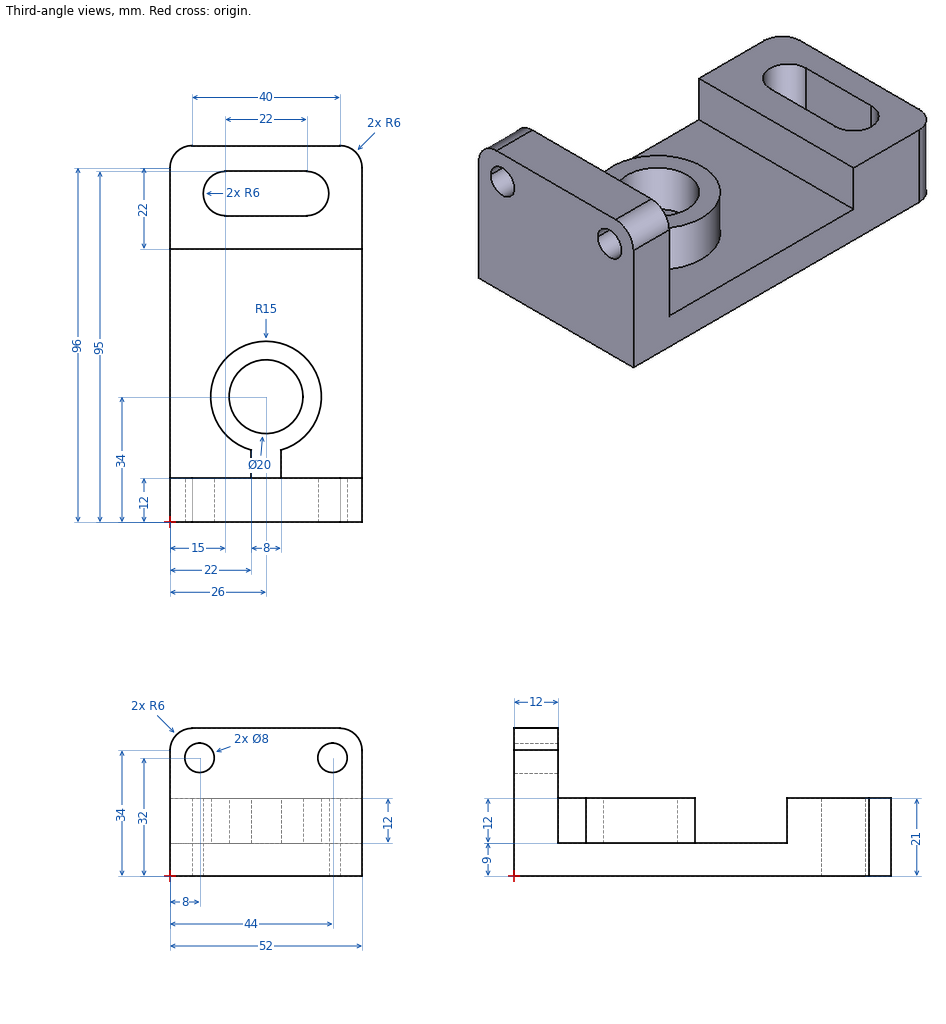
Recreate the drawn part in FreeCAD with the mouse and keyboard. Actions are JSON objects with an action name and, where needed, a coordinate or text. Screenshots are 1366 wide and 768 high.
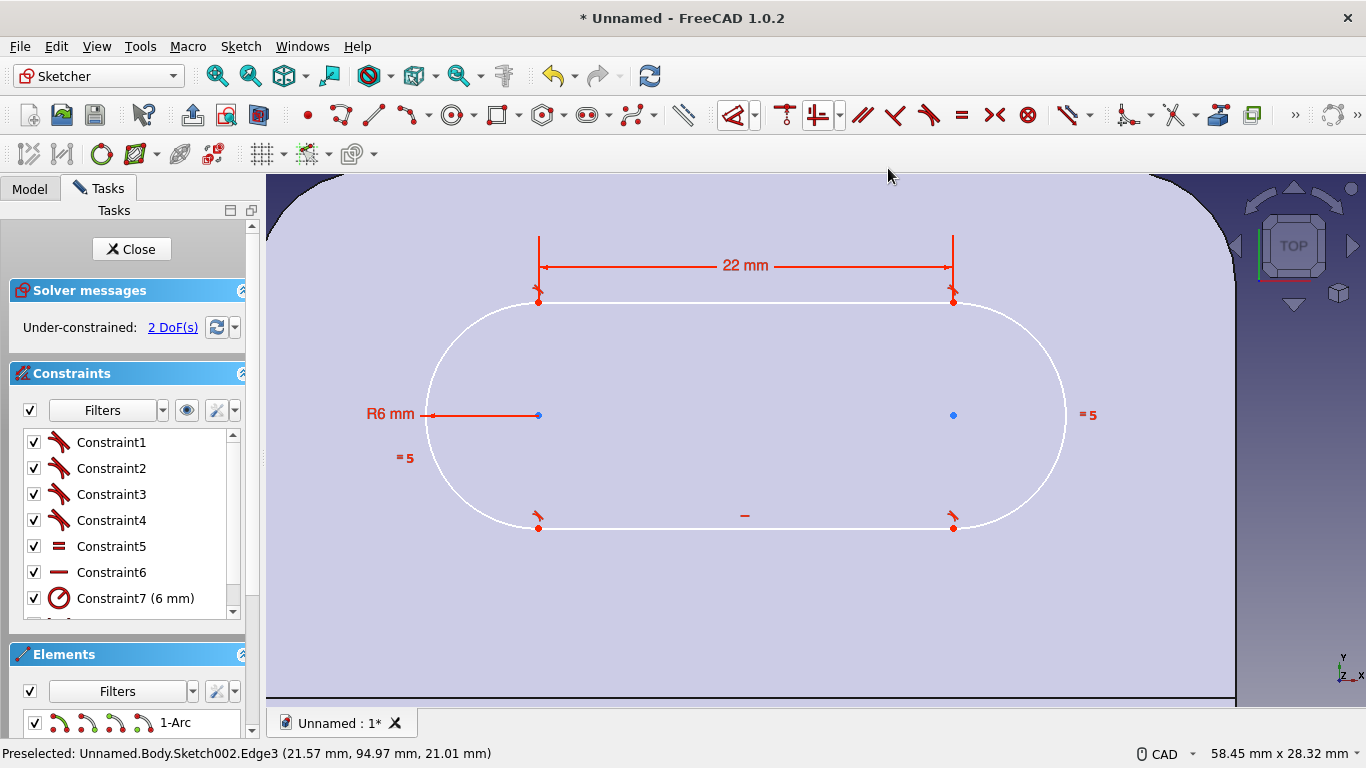
{"action": "left_click", "coordinate": [539, 303]}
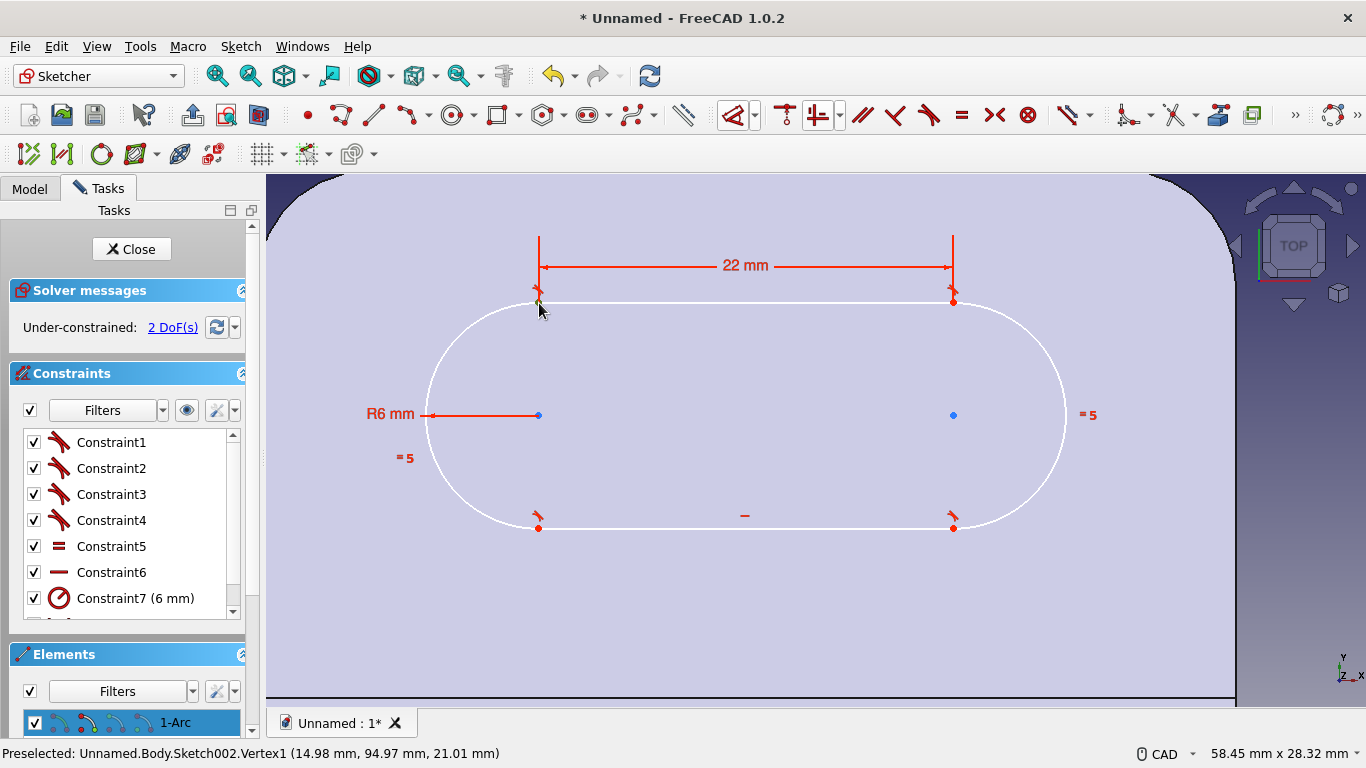
{"action": "key", "text": "l"}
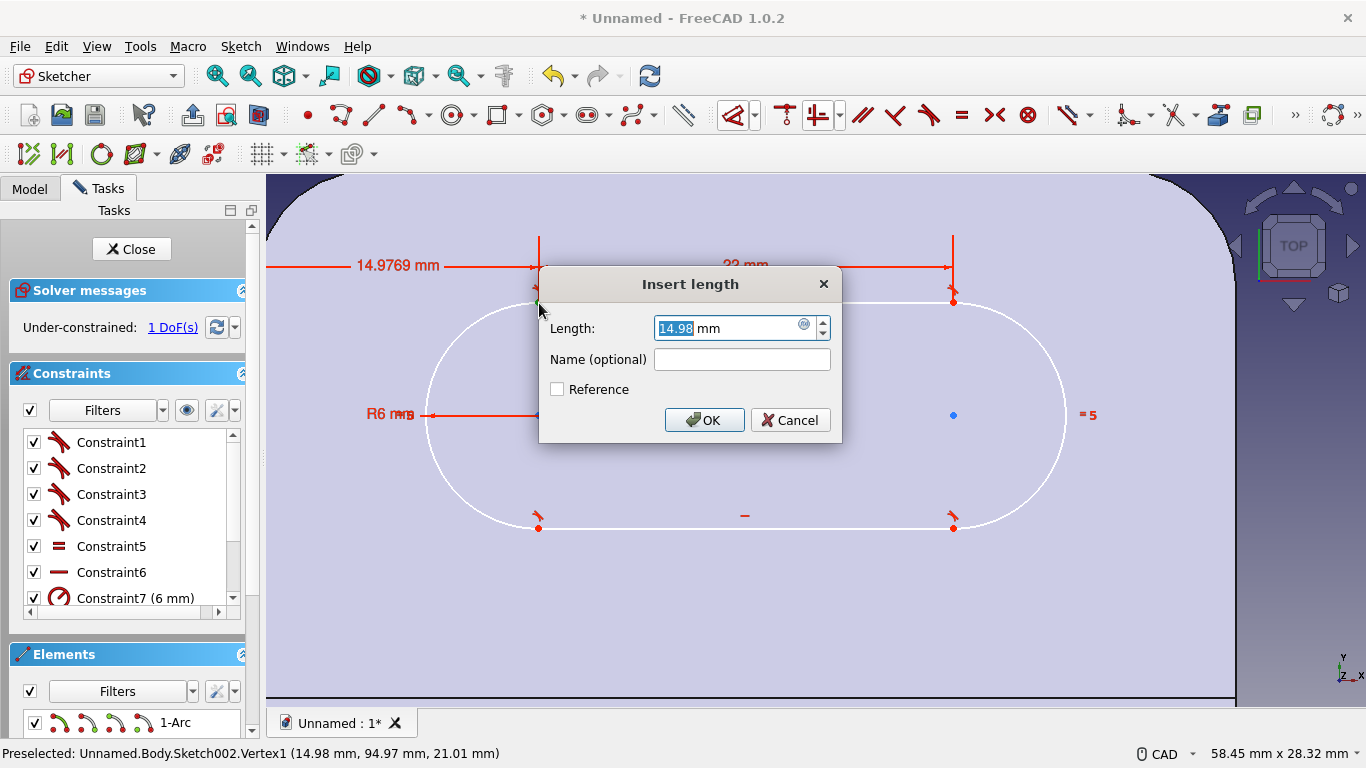
{"action": "type", "text": "15"}
{"action": "key", "text": "Return"}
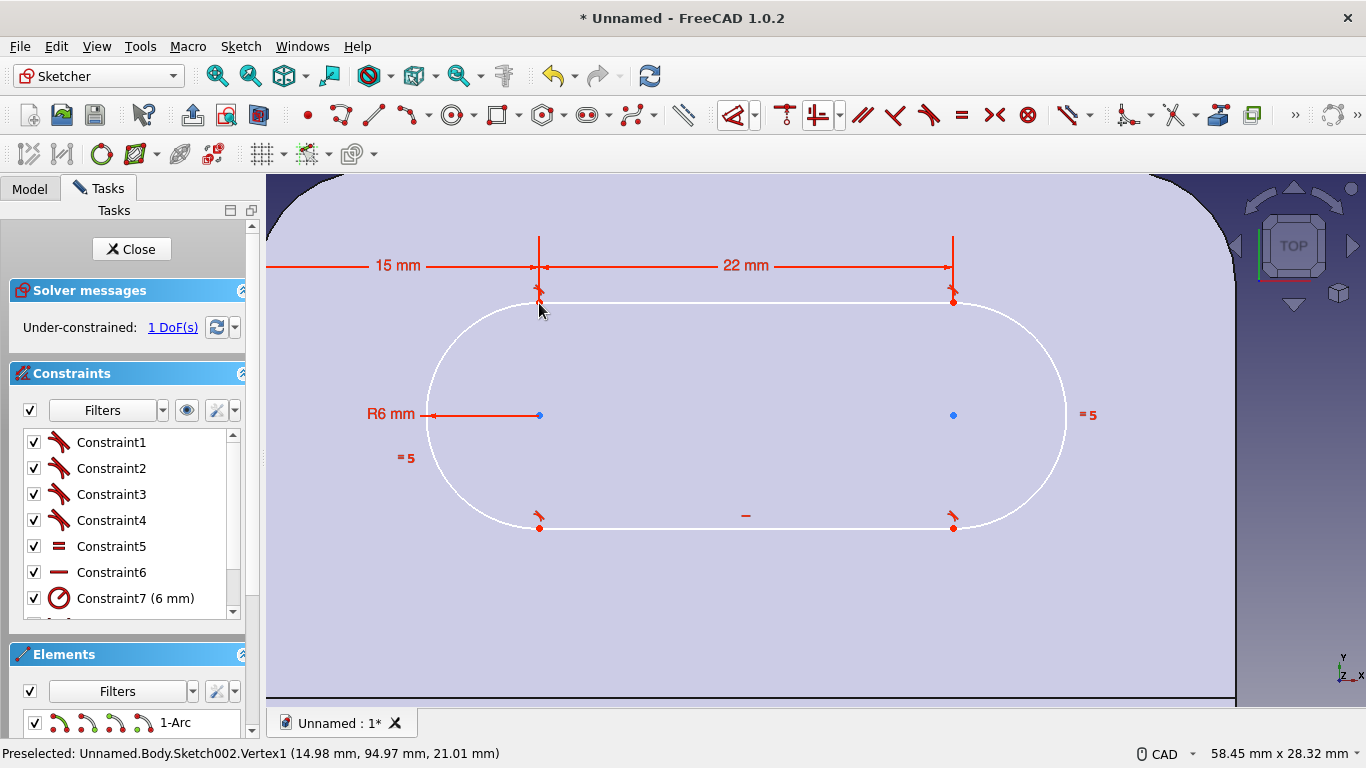
{"action": "left_click", "coordinate": [539, 303]}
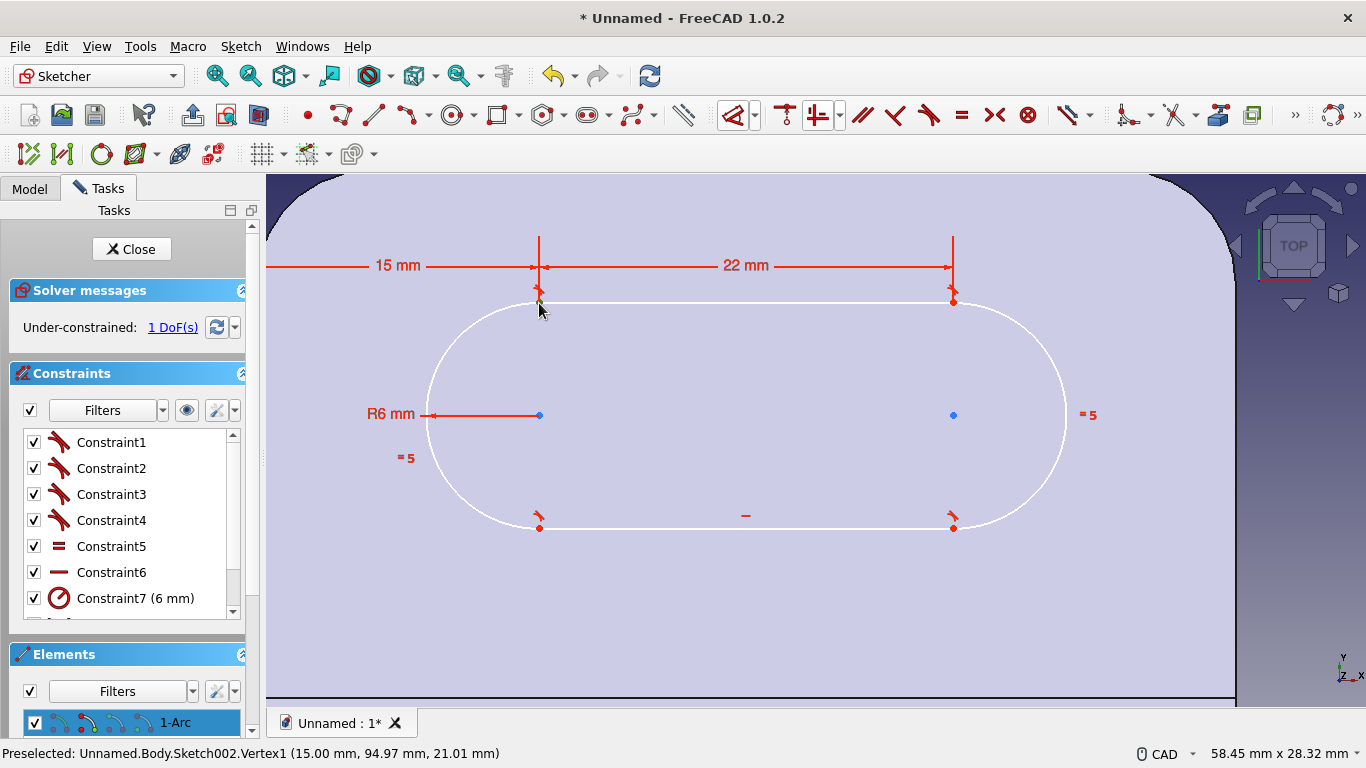
{"action": "key", "text": "i"}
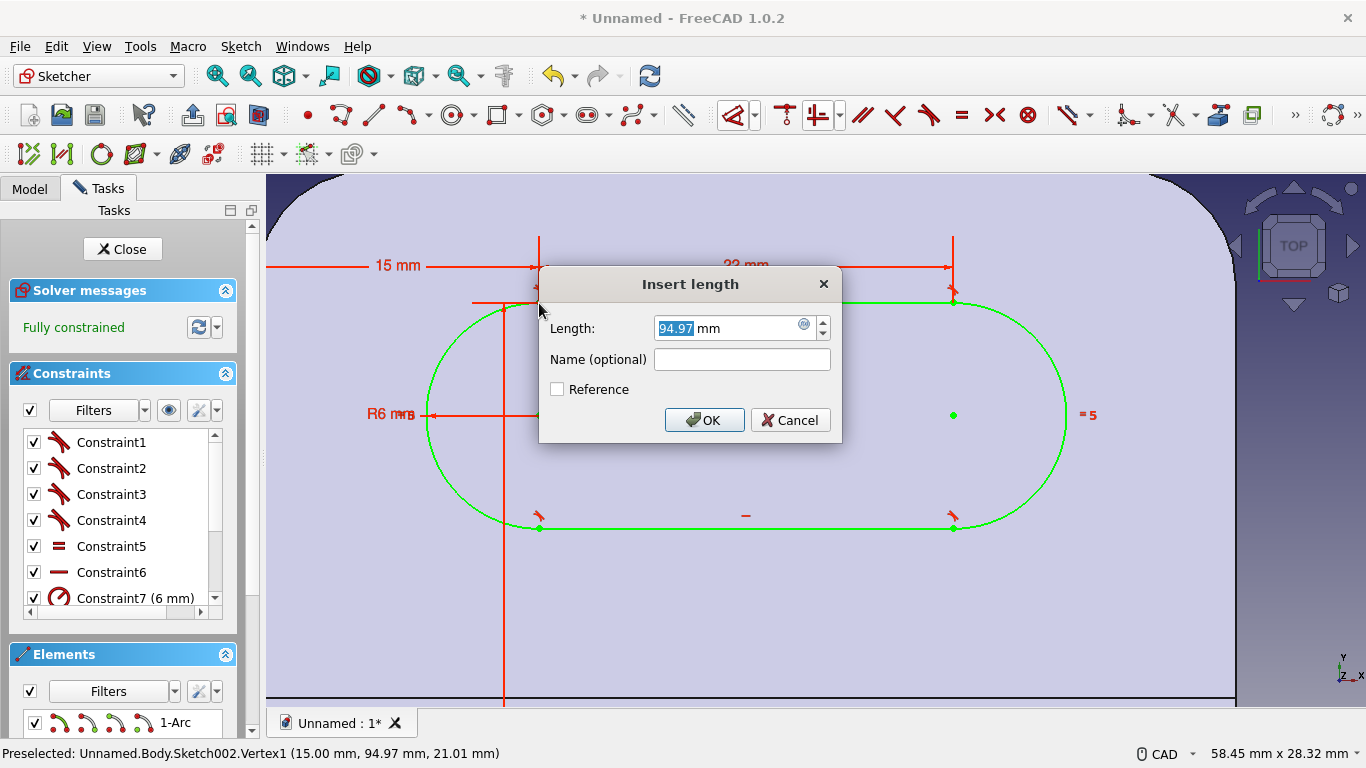
{"action": "type", "text": "95"}
{"action": "key", "text": "Return"}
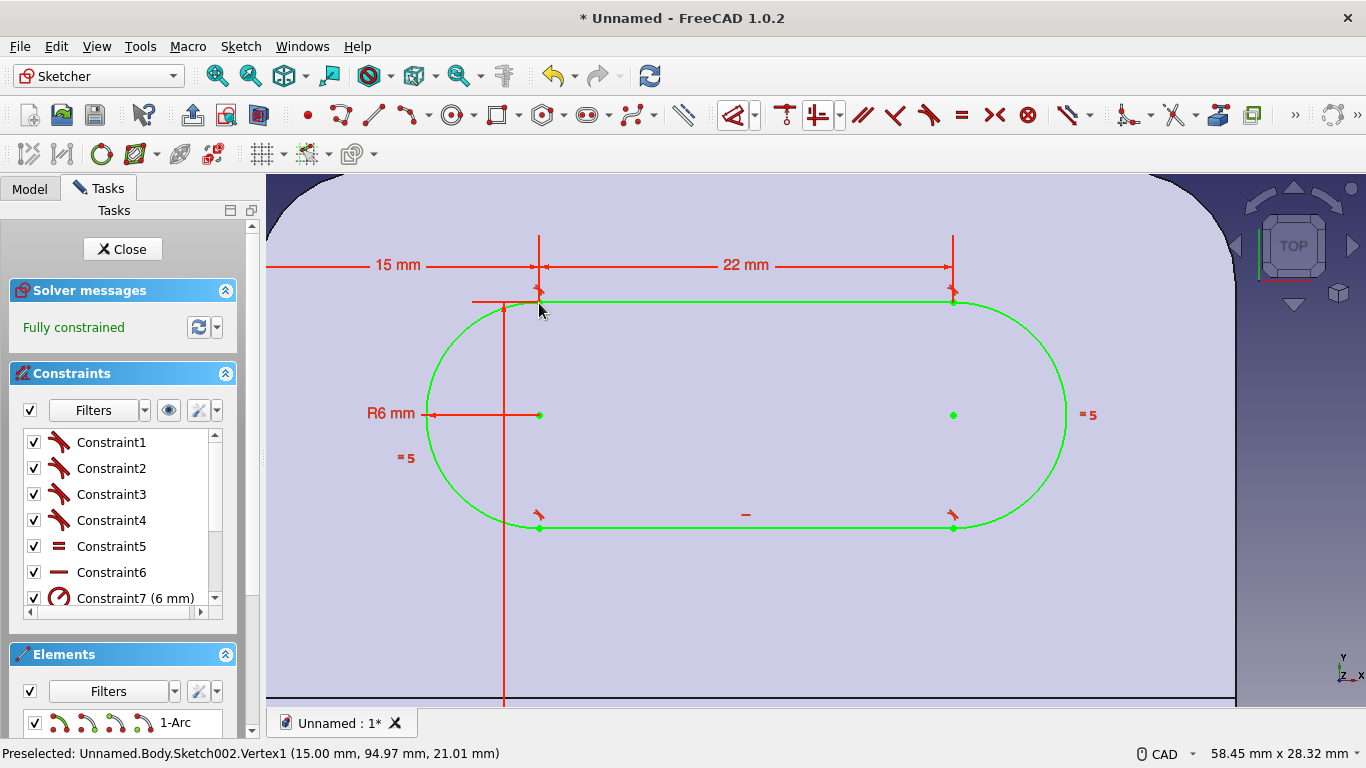
{"action": "left_click", "coordinate": [123, 249]}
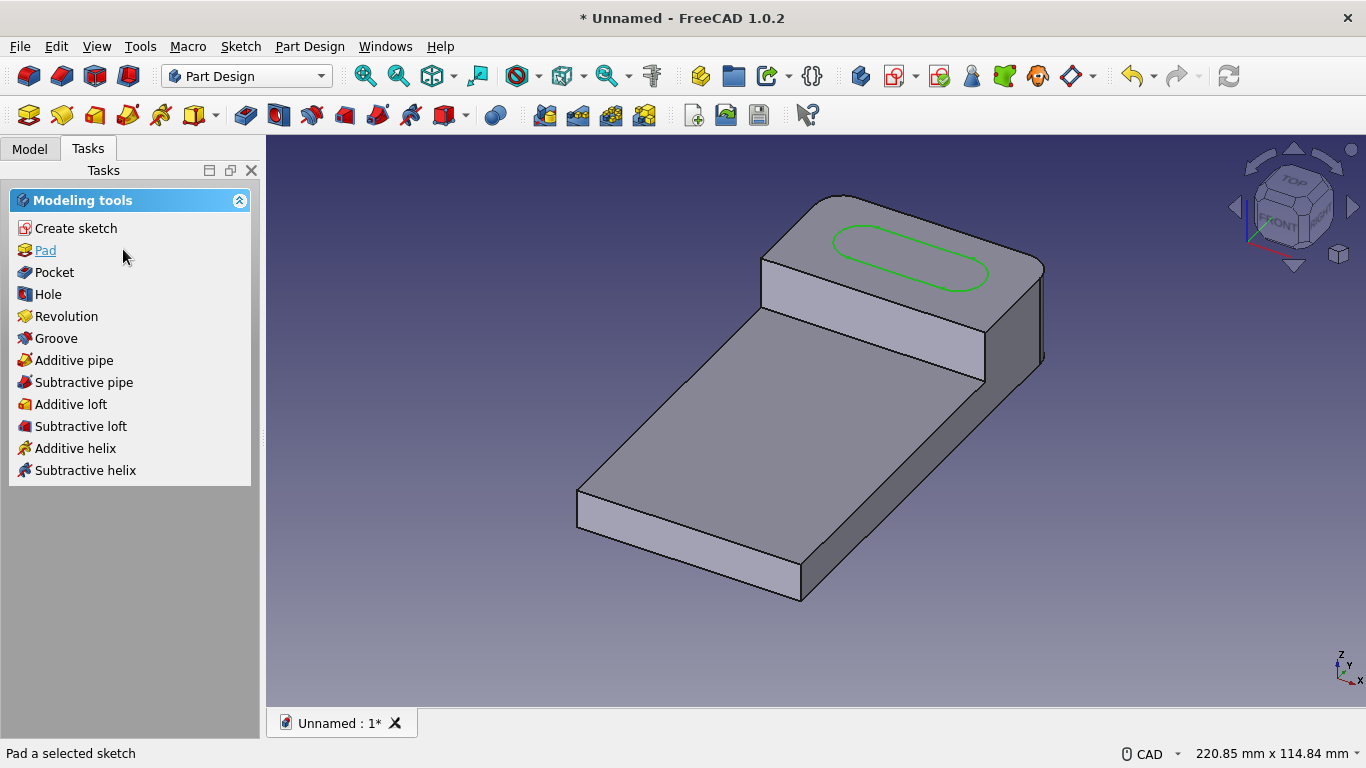
{"action": "left_click", "coordinate": [246, 116]}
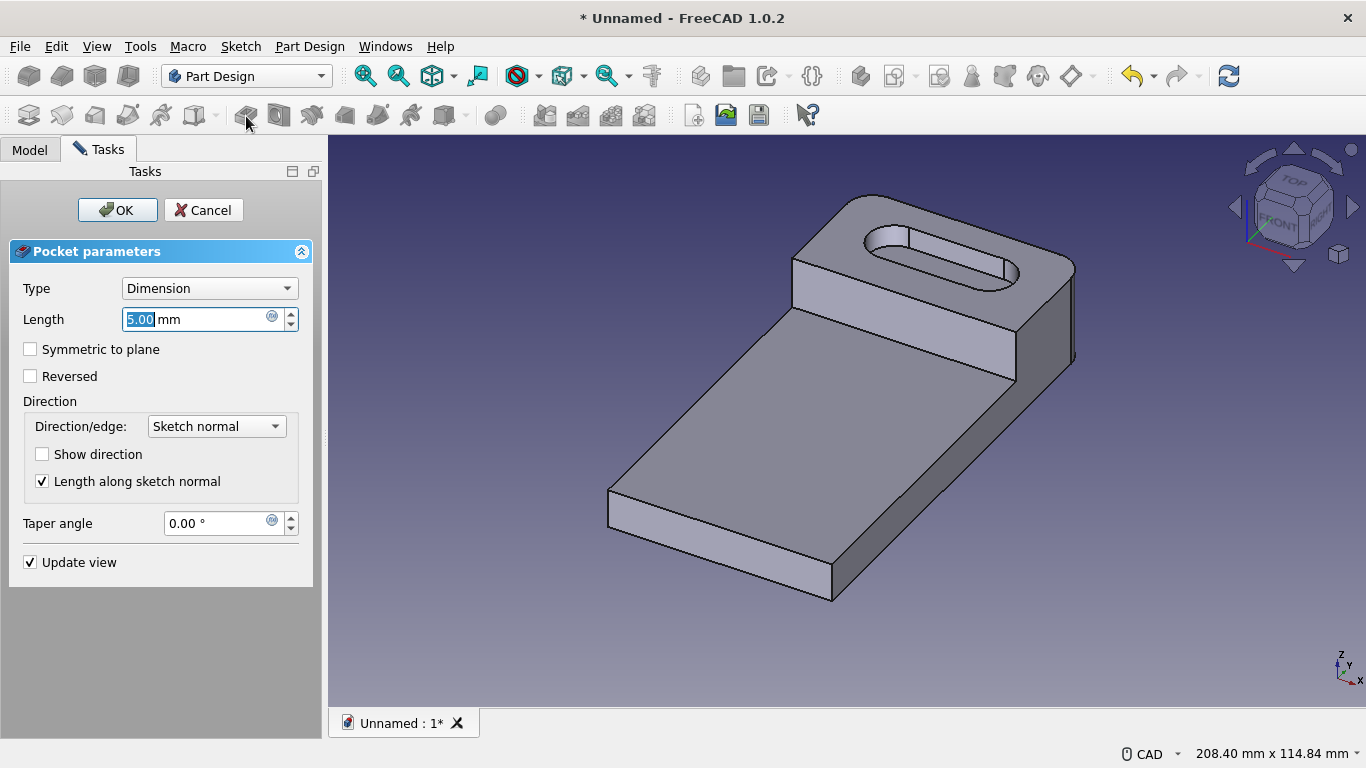
{"action": "type", "text": "21"}
{"action": "key", "text": "Tab"}